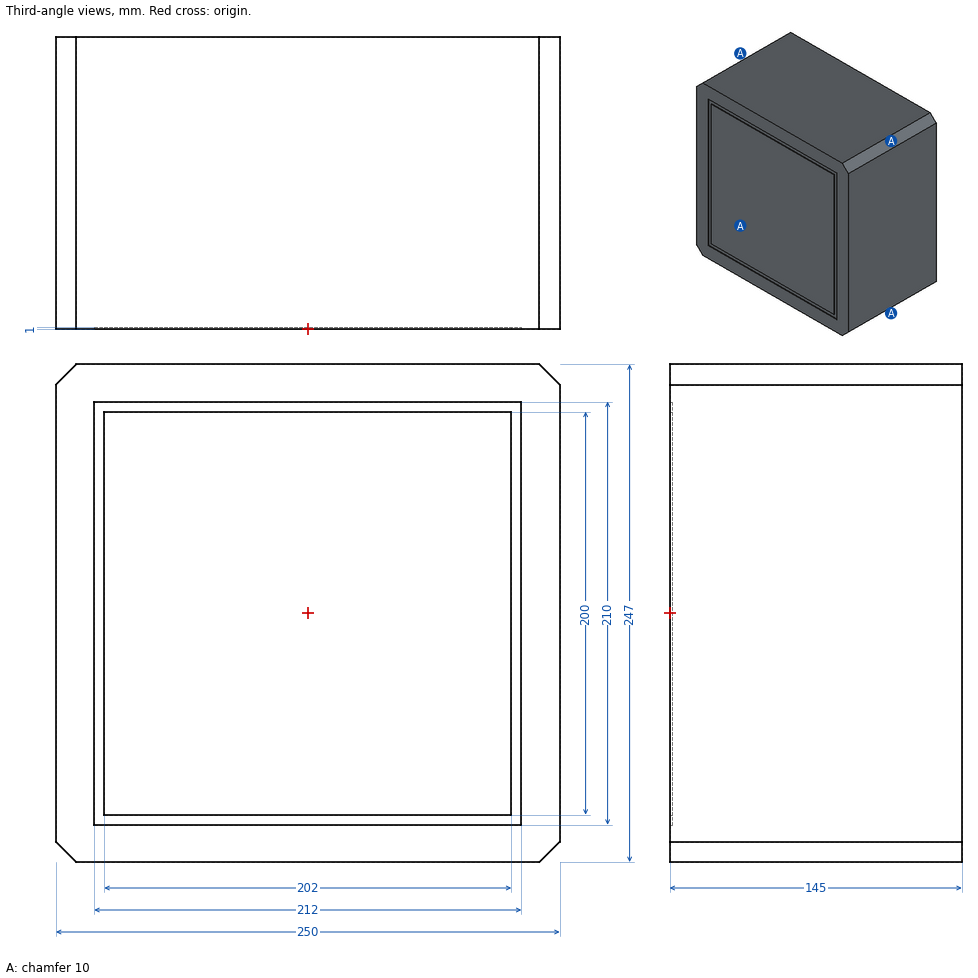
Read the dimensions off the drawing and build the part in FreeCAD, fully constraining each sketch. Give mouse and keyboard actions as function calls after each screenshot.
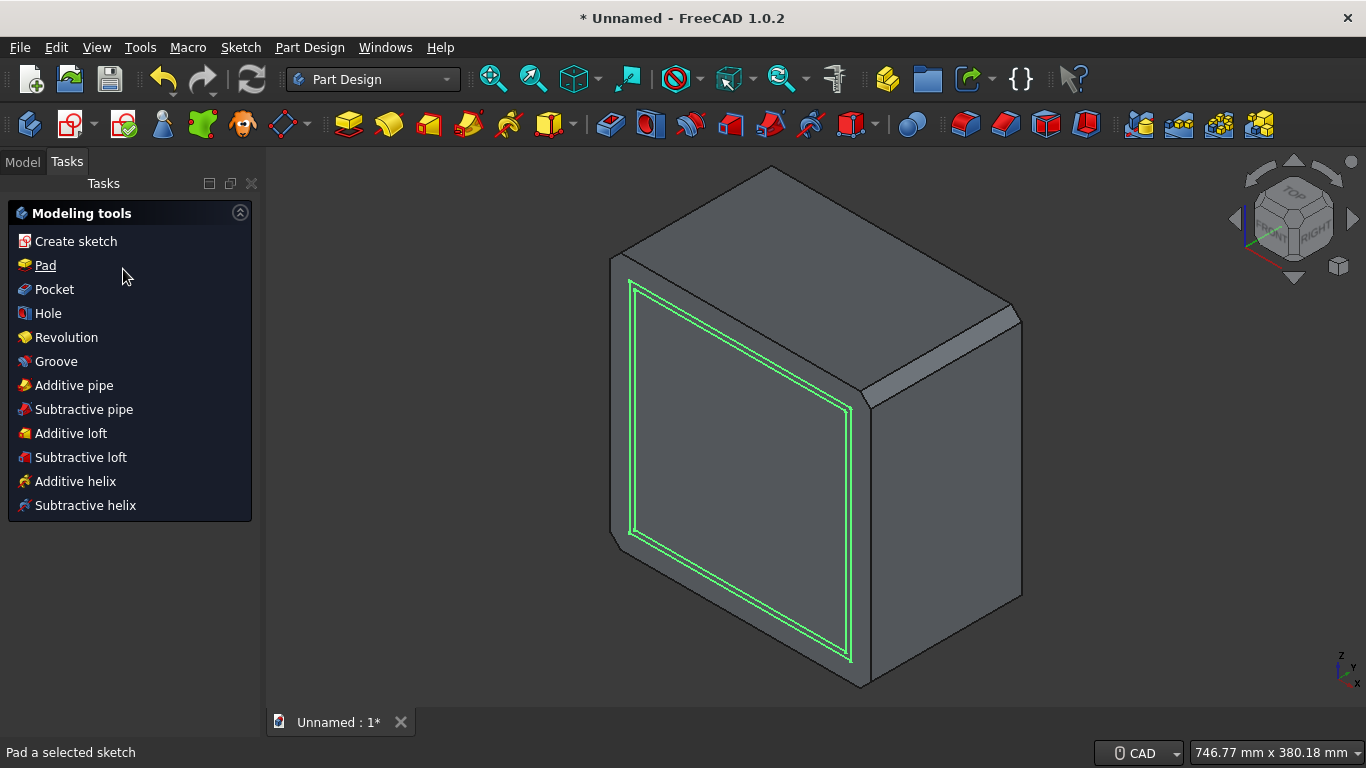
click(612, 124)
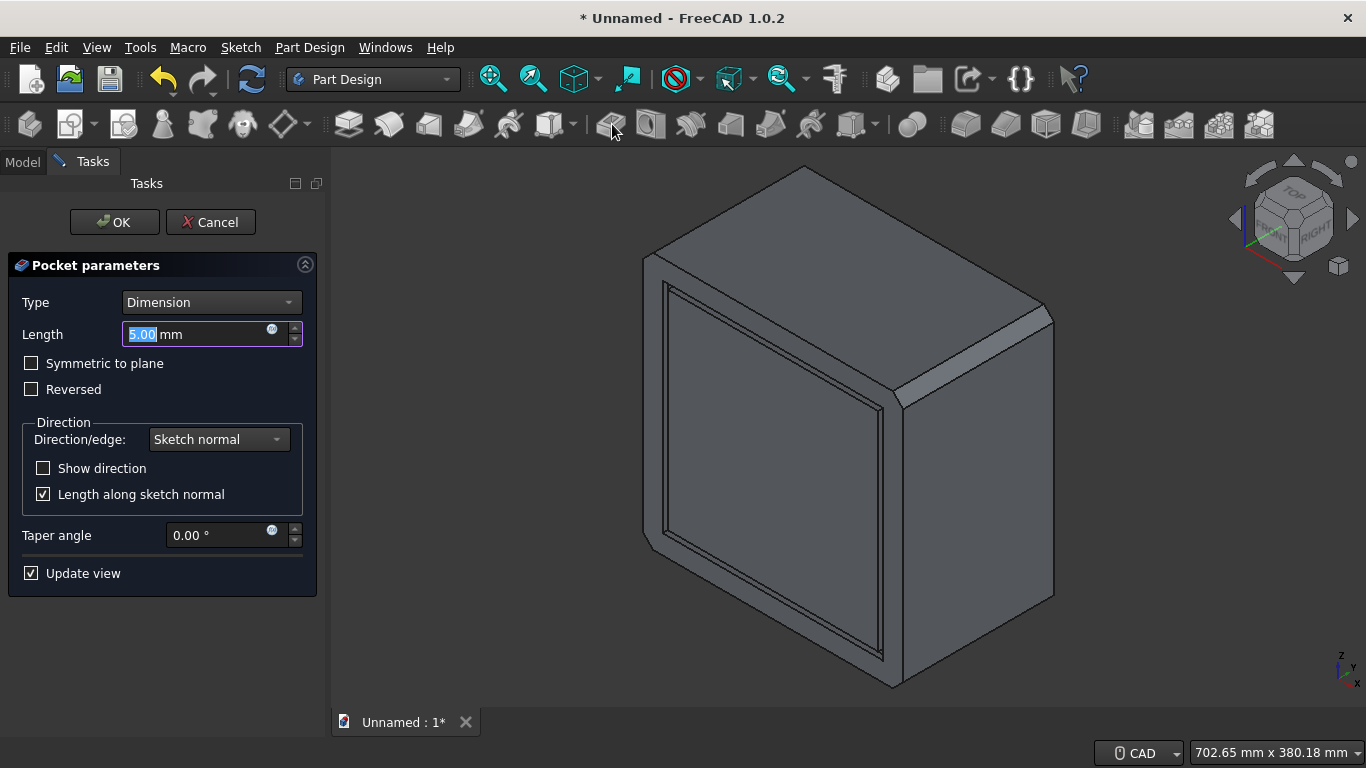
text(1)
key(Tab)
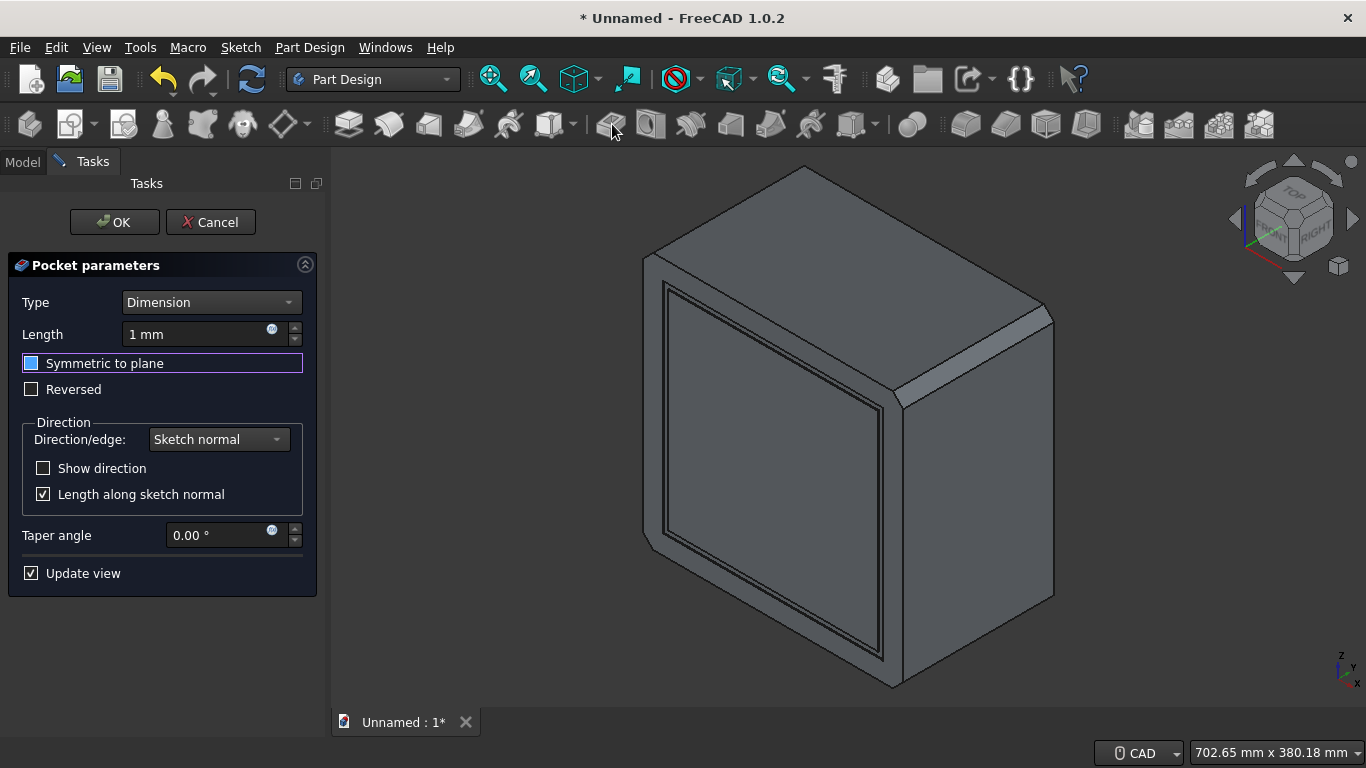
click(115, 222)